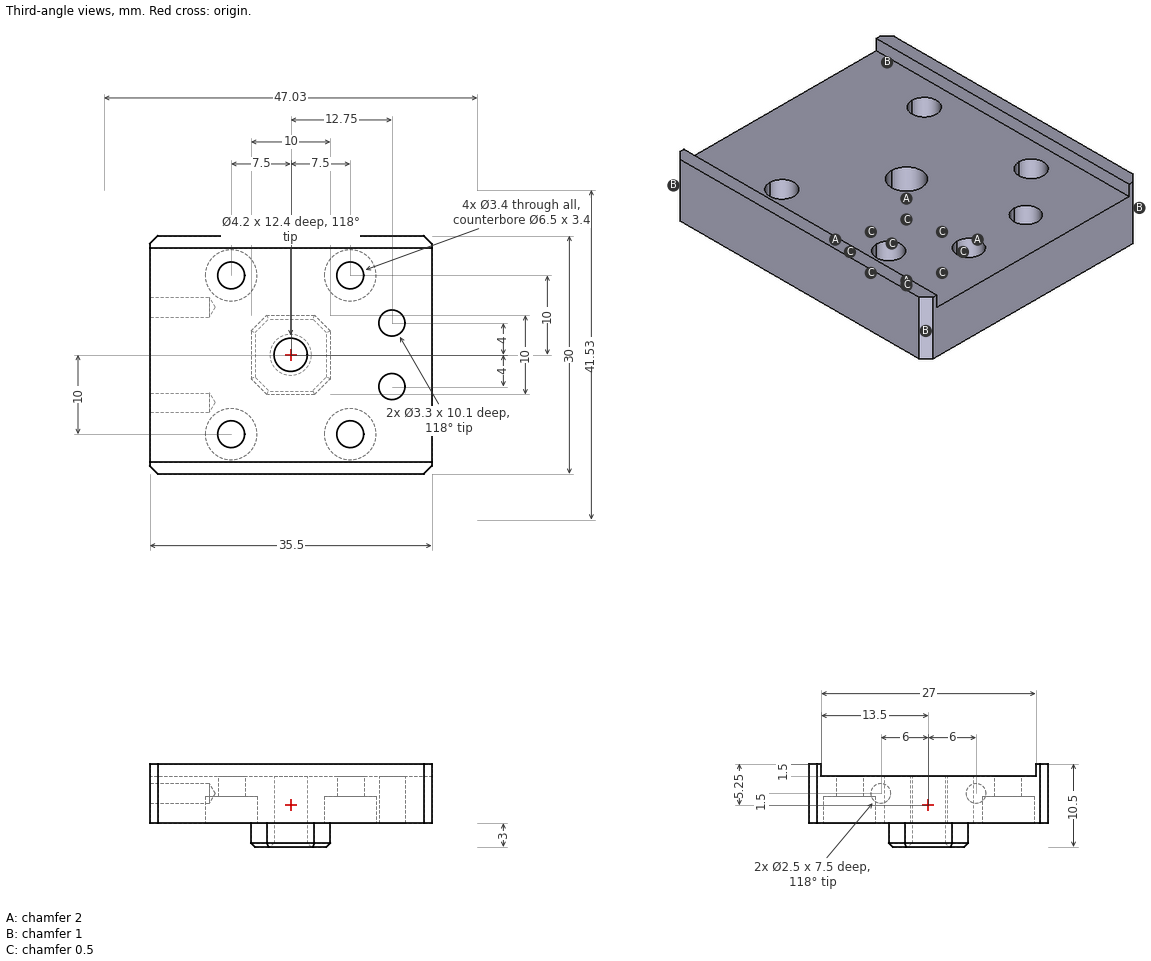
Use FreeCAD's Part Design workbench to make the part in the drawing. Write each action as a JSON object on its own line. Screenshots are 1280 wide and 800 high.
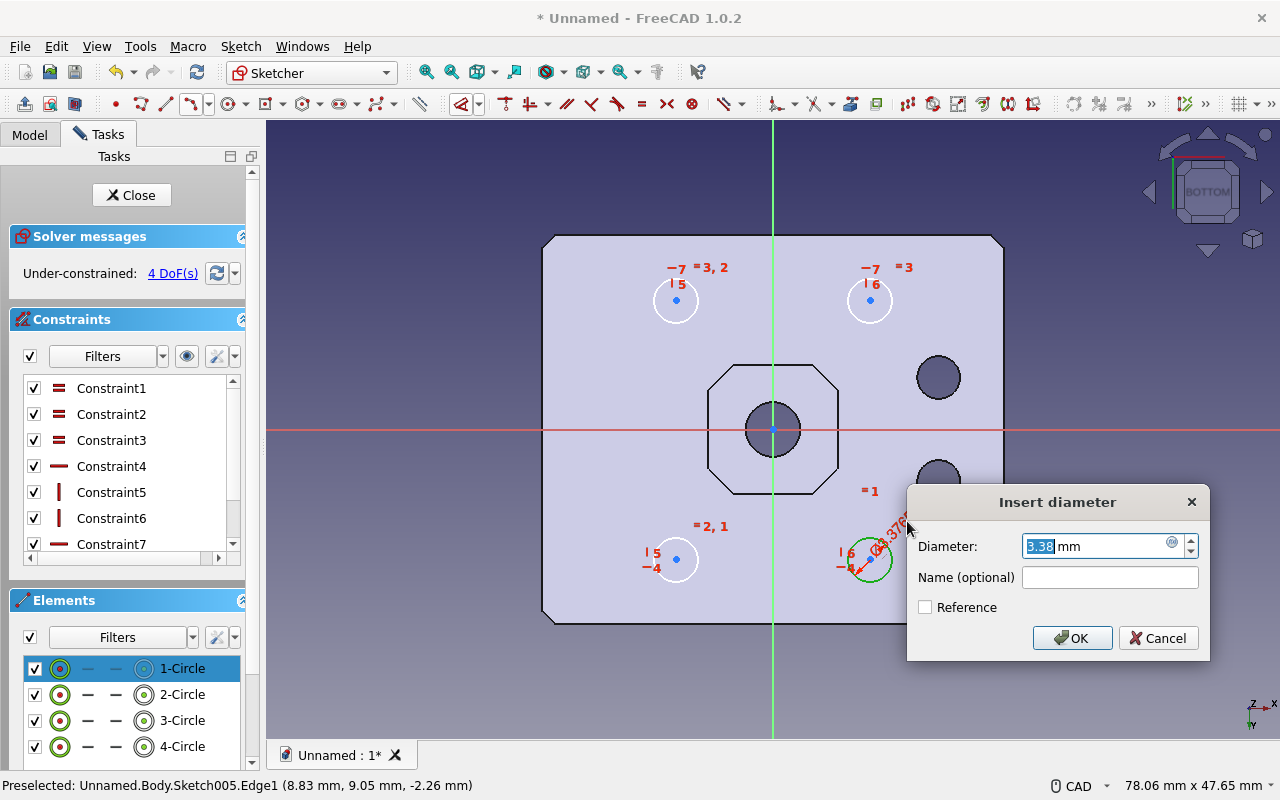
{"action": "type", "text": "3.4"}
{"action": "key", "text": "Return"}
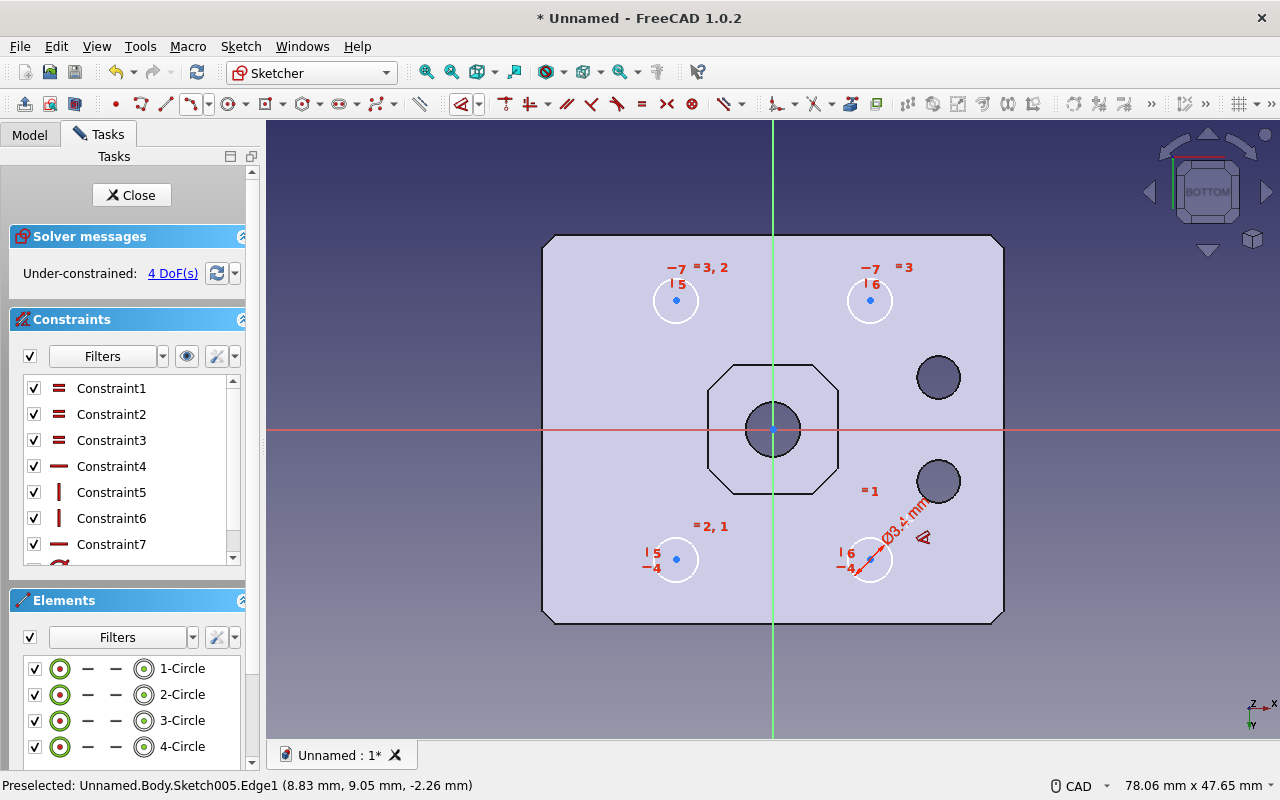
{"action": "left_click", "coordinate": [870, 560]}
{"action": "left_click", "coordinate": [904, 495]}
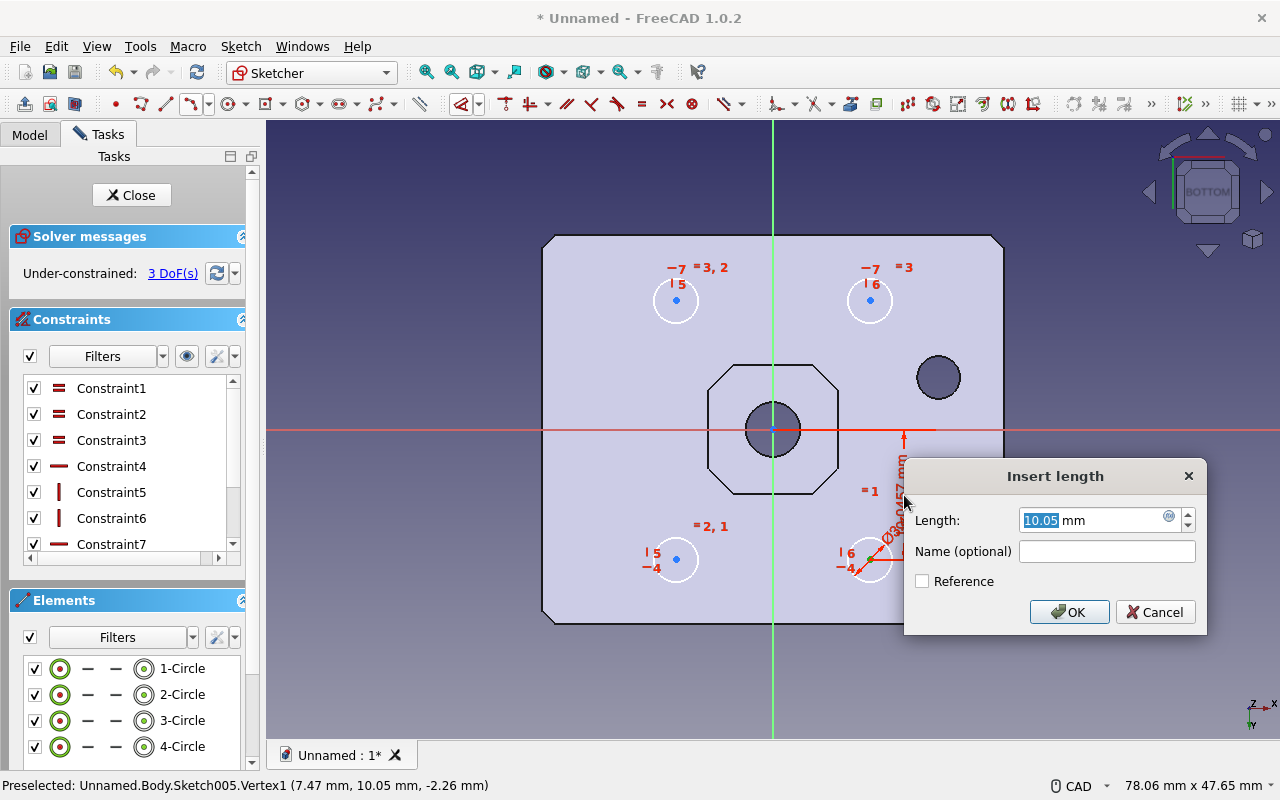
{"action": "type", "text": "10"}
{"action": "key", "text": "Return"}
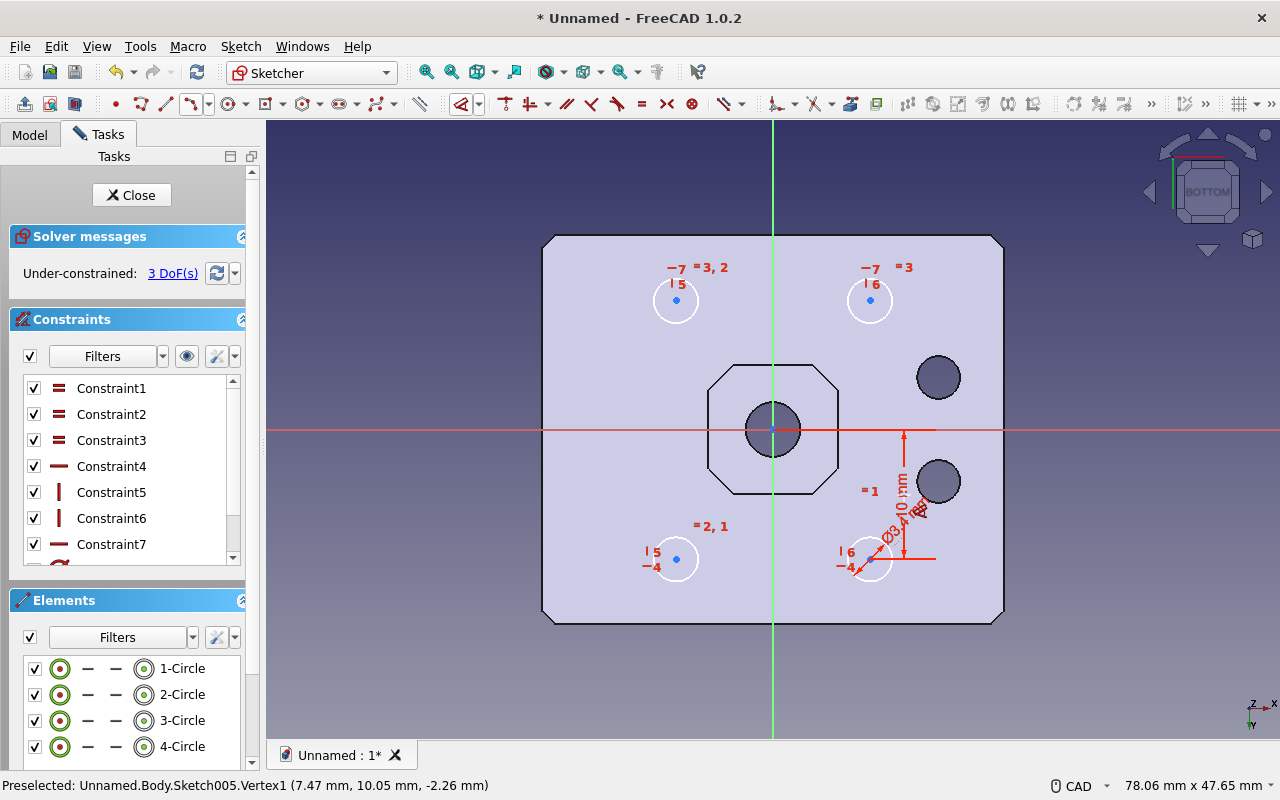
{"action": "left_click", "coordinate": [676, 301]}
{"action": "left_click", "coordinate": [642, 365]}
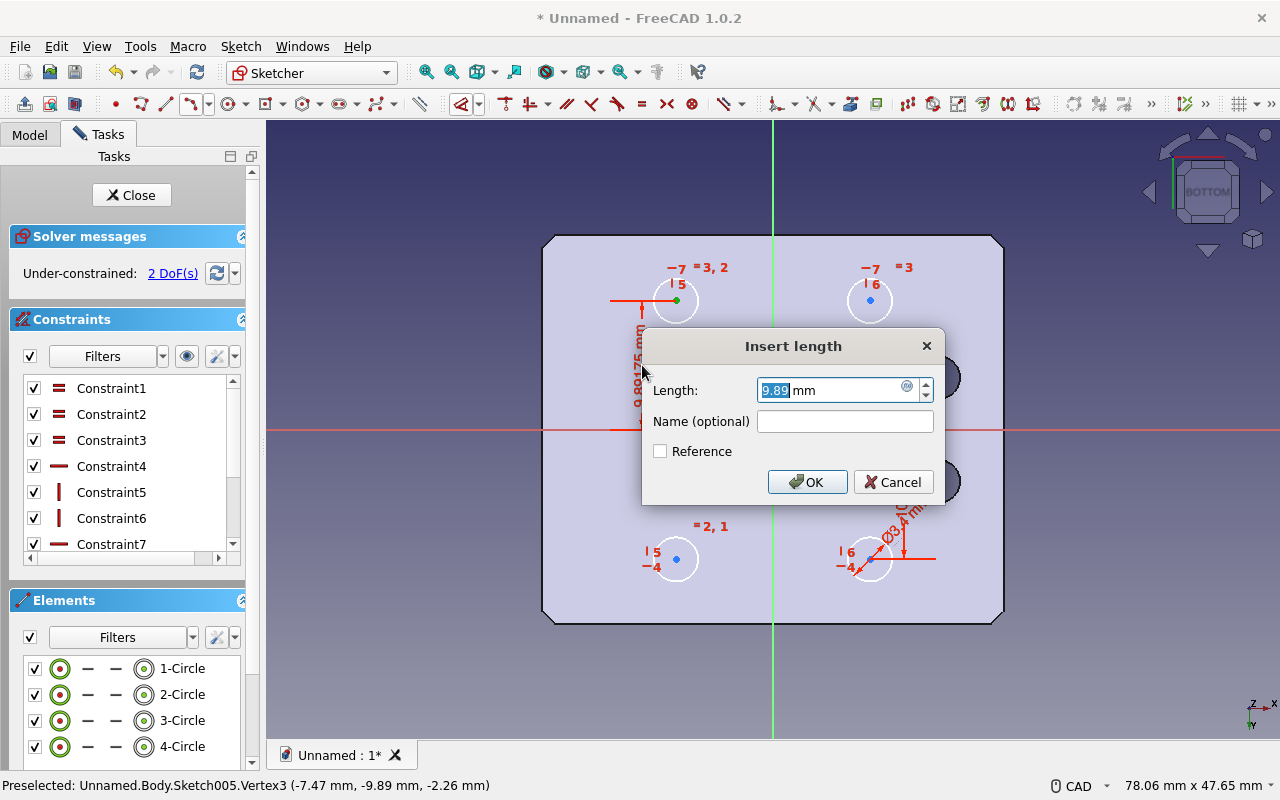
{"action": "type", "text": "10"}
{"action": "key", "text": "Return"}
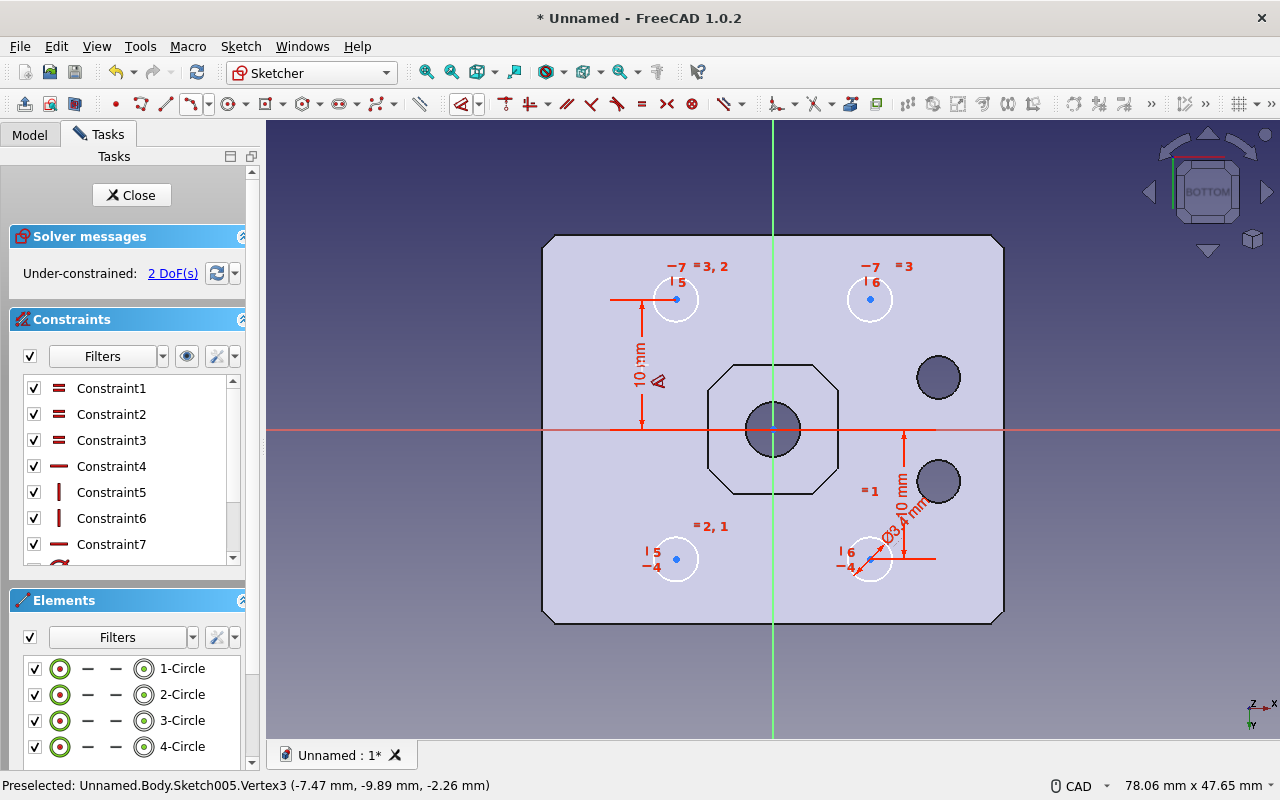
{"action": "left_click", "coordinate": [870, 559]}
{"action": "left_click", "coordinate": [821, 593]}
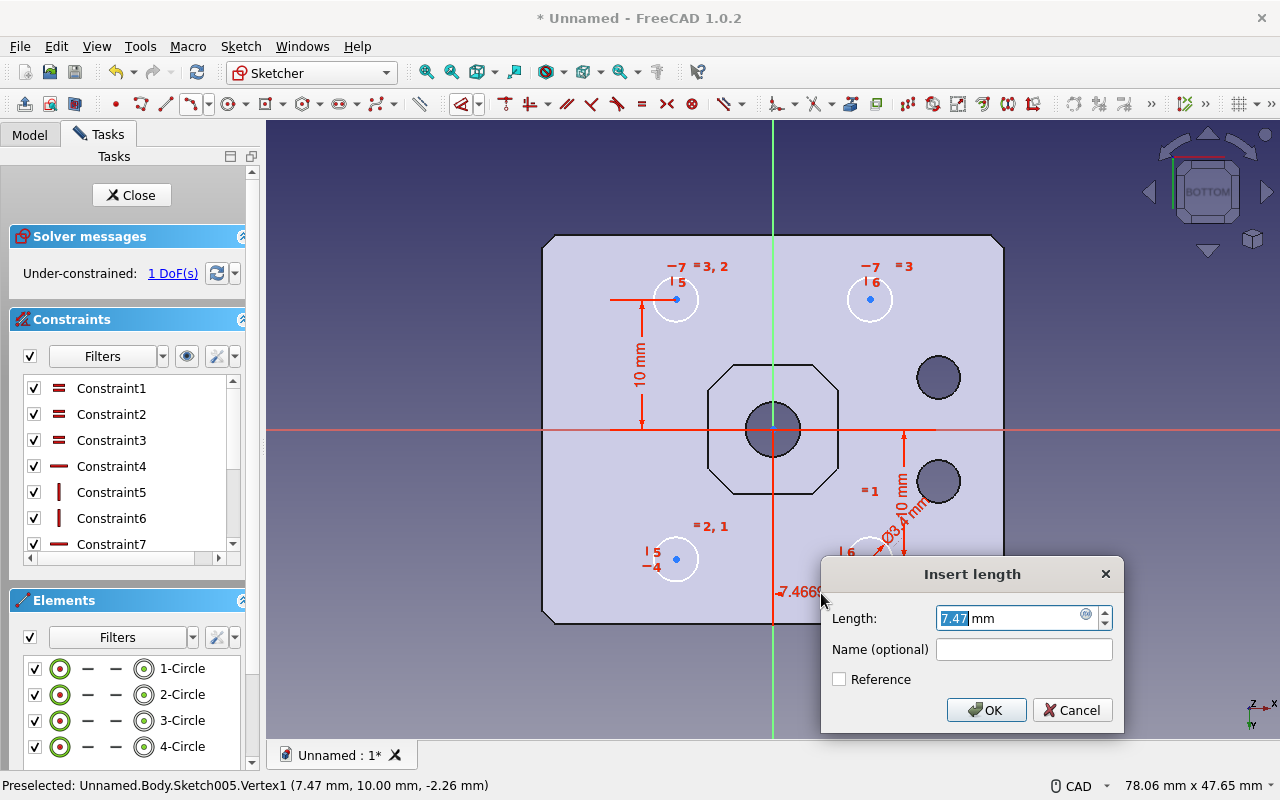
{"action": "type", "text": "7.5"}
{"action": "key", "text": "Return"}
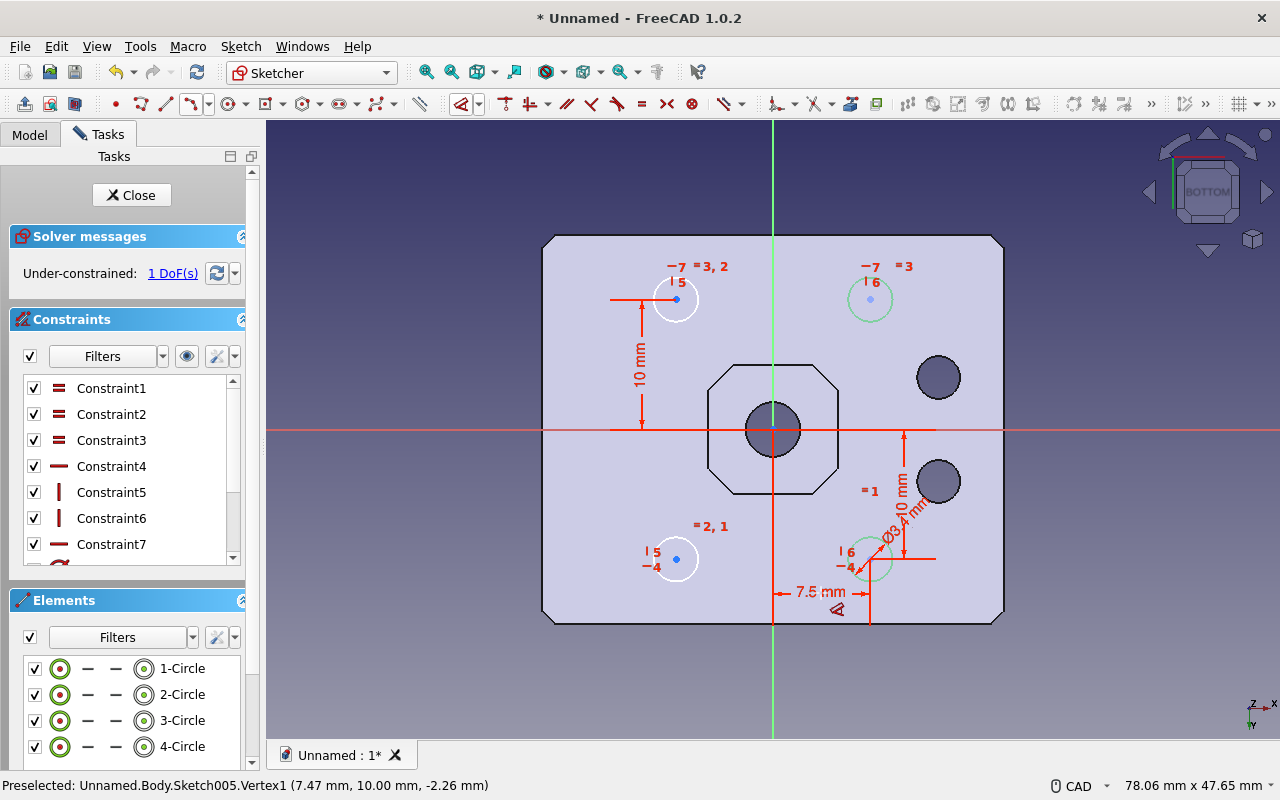
{"action": "left_click", "coordinate": [676, 559]}
{"action": "left_click", "coordinate": [725, 593]}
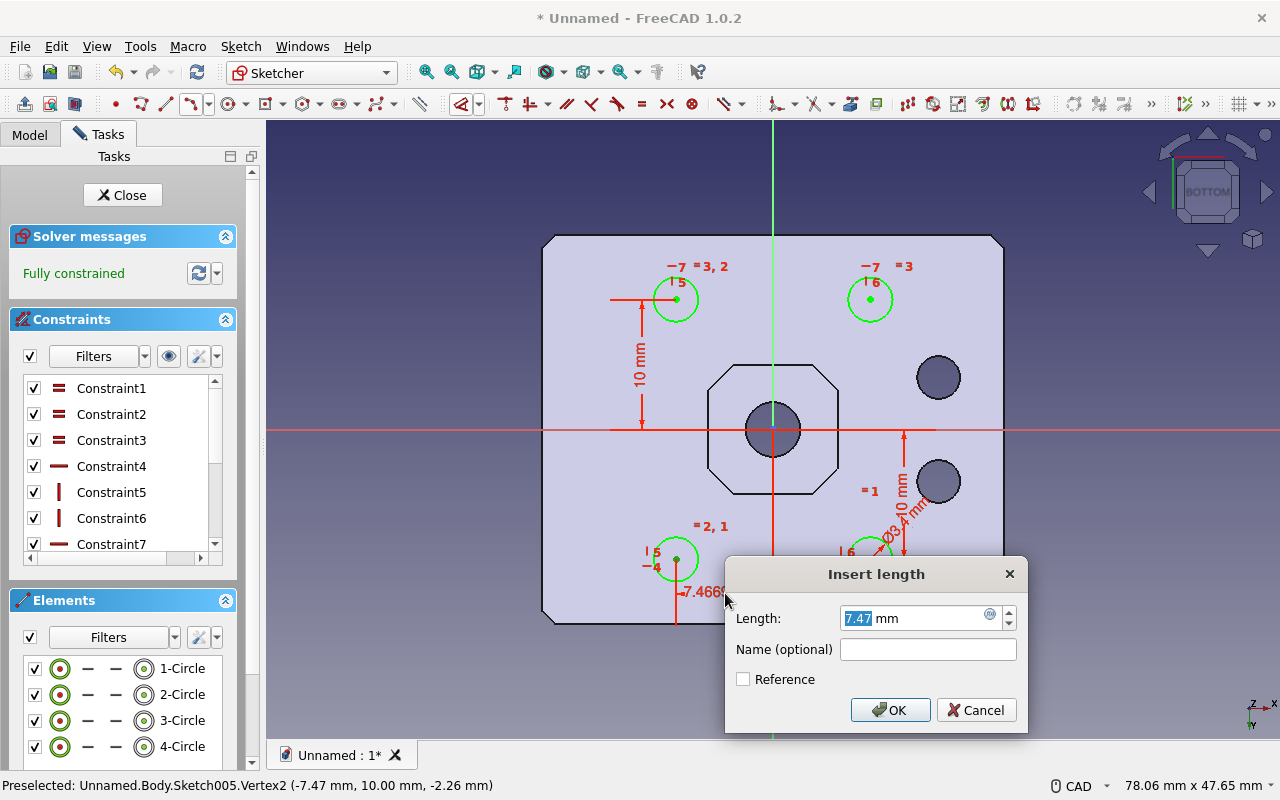
{"action": "type", "text": "7.5"}
{"action": "key", "text": "Return"}
{"action": "key", "text": "Escape"}